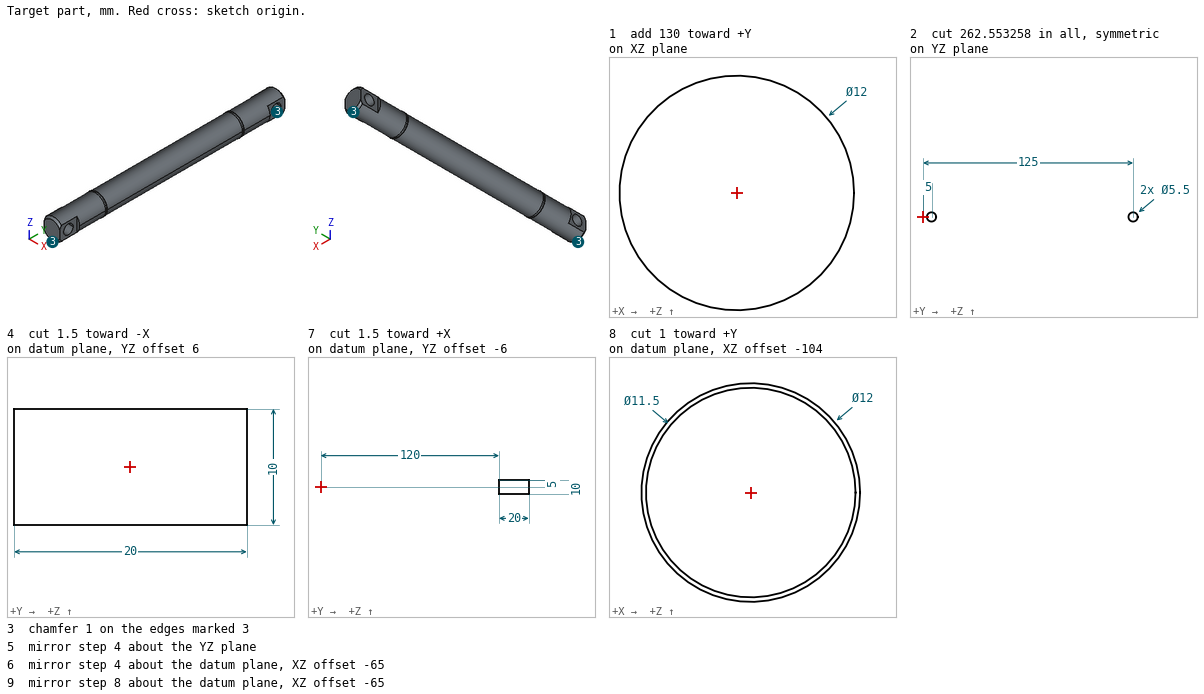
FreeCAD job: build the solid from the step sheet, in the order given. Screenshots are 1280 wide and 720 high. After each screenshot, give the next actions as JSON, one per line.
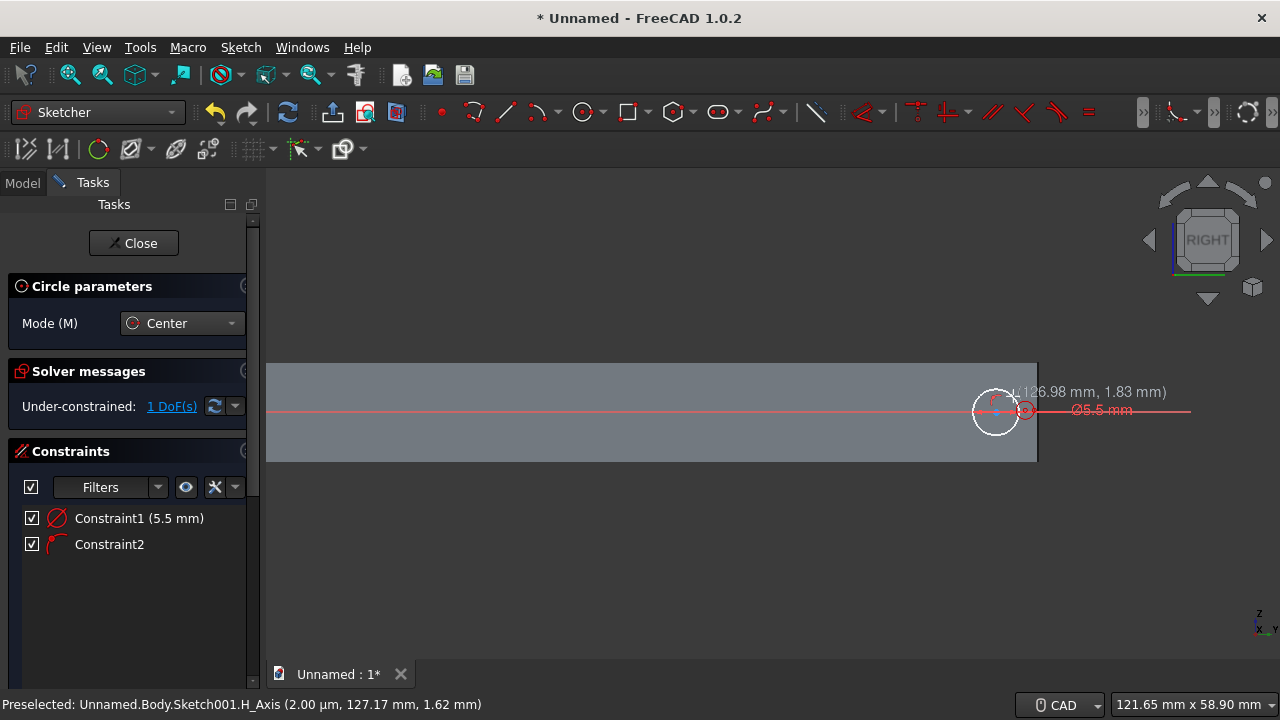
{"action": "scroll", "coordinate": [969, 415], "scroll_direction": "down", "scroll_amount": 3}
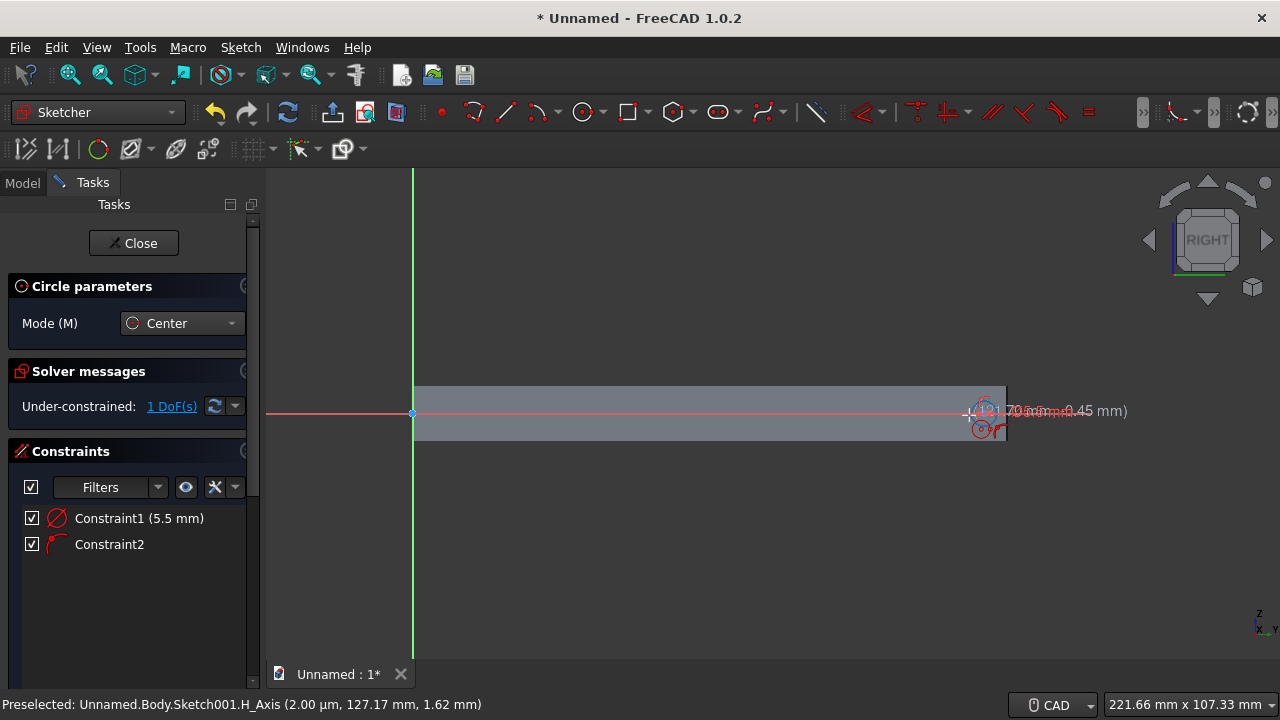
{"action": "scroll", "coordinate": [435, 414], "scroll_direction": "up", "scroll_amount": 3}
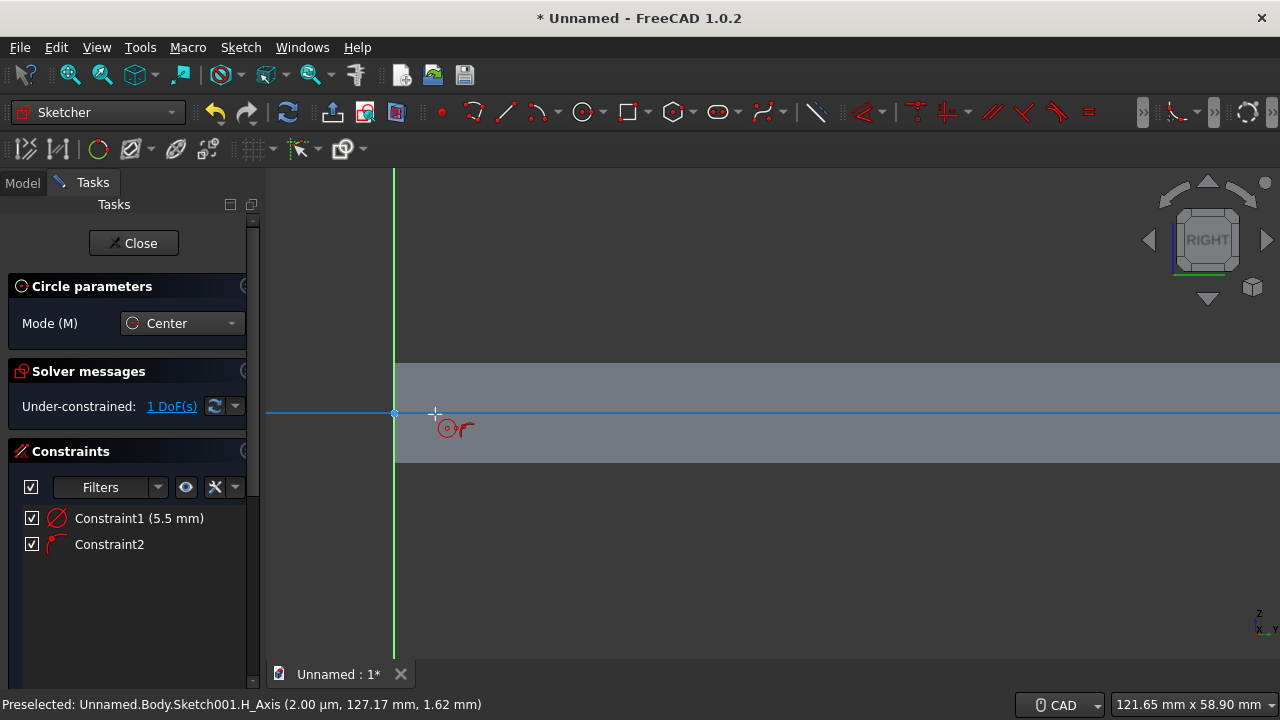
{"action": "left_click", "coordinate": [436, 413]}
{"action": "mouse_move", "coordinate": [452, 397]}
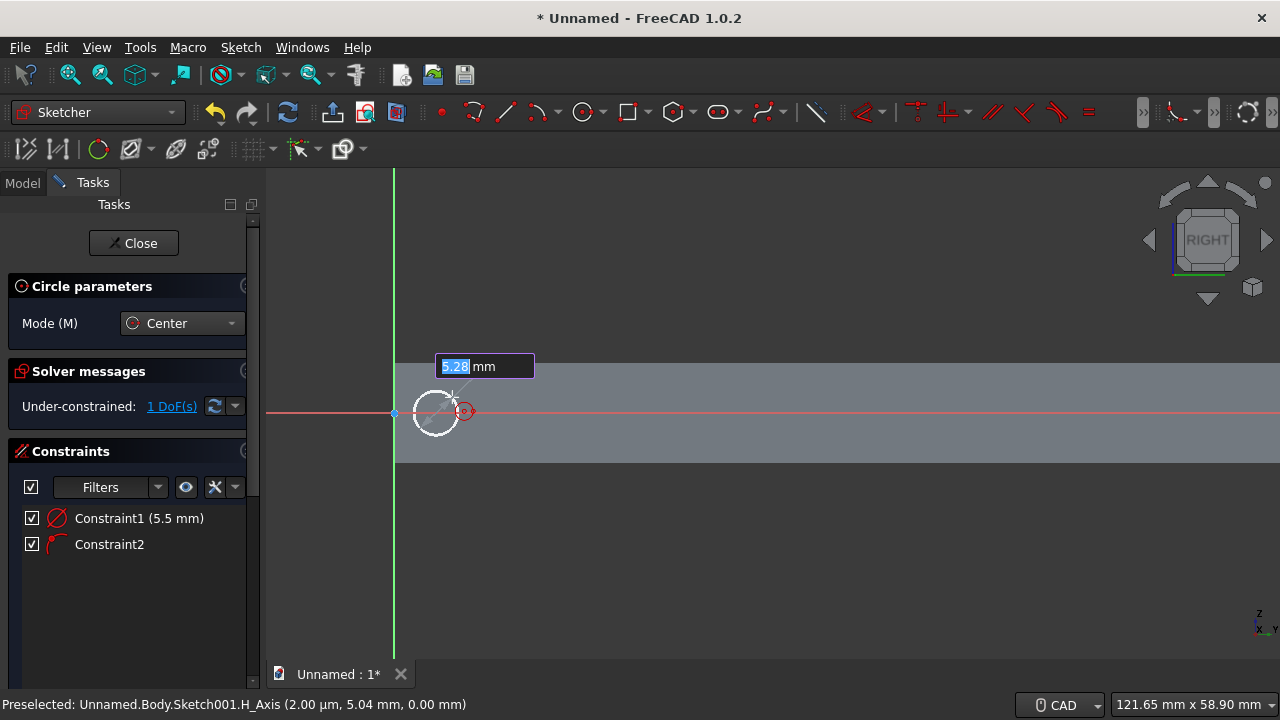
{"action": "type", "text": "5.5"}
{"action": "key", "text": "Return"}
{"action": "key", "text": "Escape"}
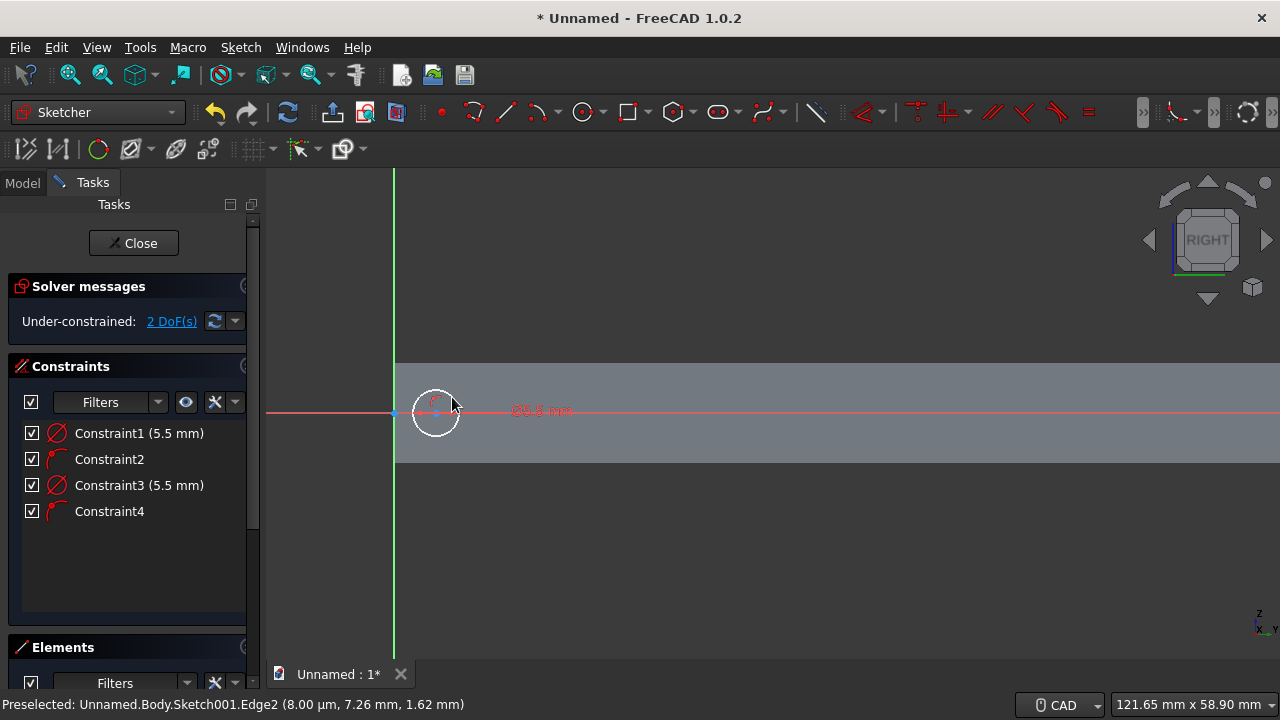
{"action": "key", "text": "d"}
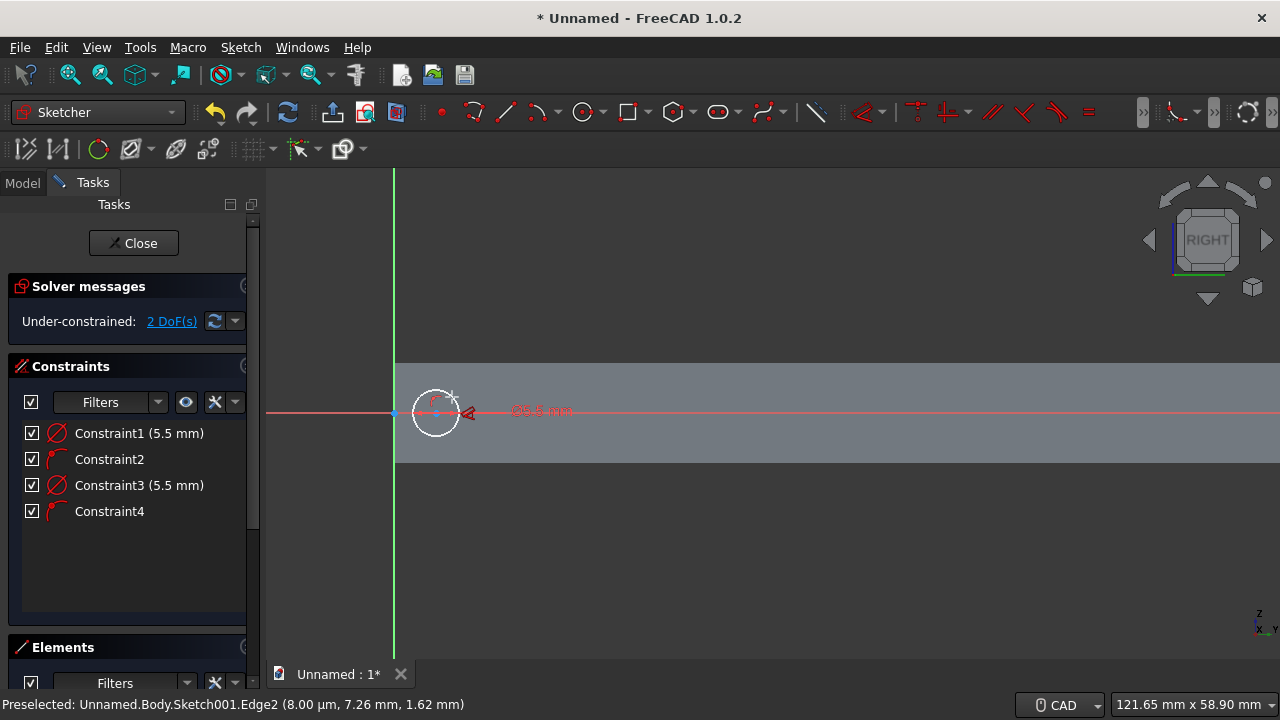
{"action": "left_click", "coordinate": [436, 413]}
{"action": "left_click", "coordinate": [415, 447]}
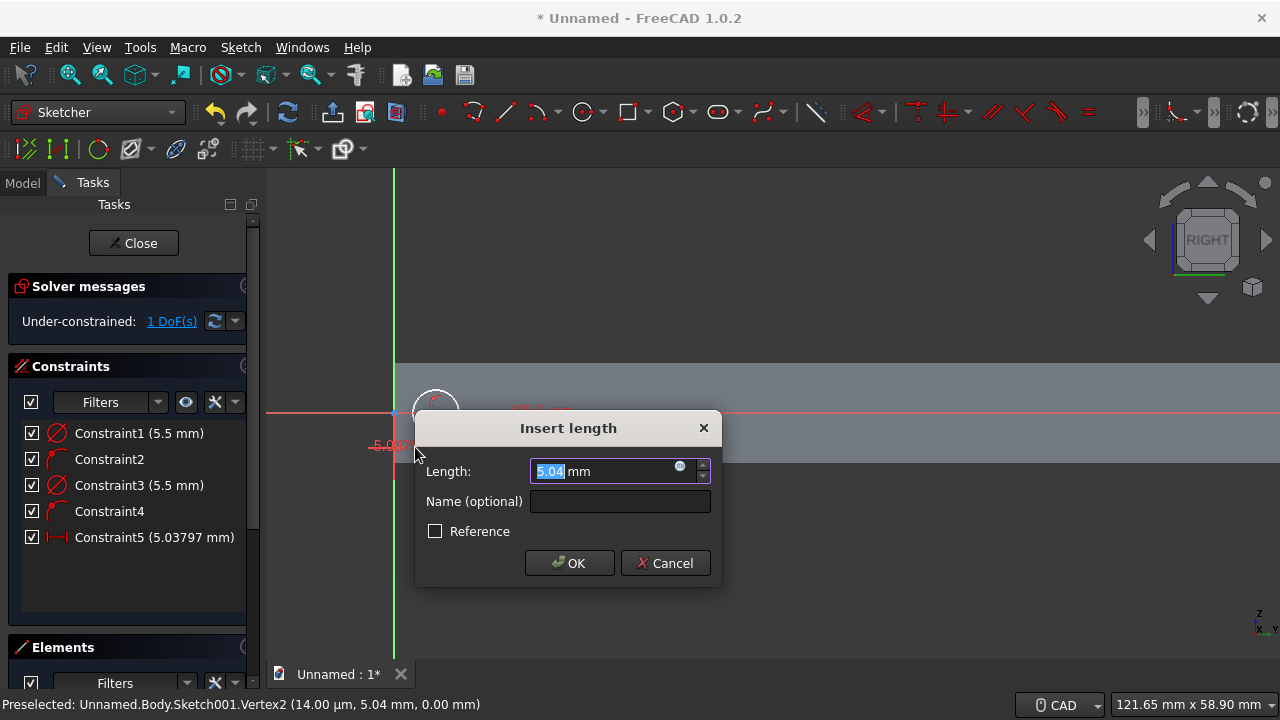
{"action": "type", "text": "5"}
{"action": "key", "text": "Return"}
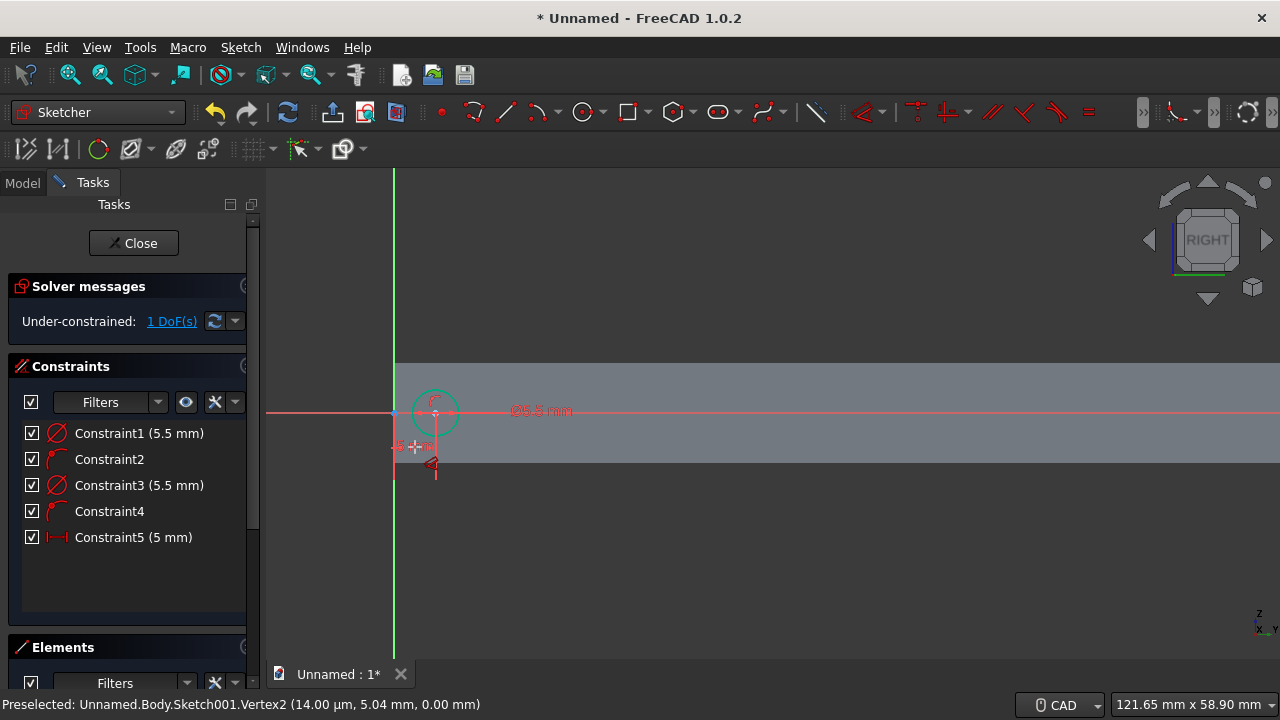
{"action": "scroll", "coordinate": [435, 414], "scroll_direction": "down", "scroll_amount": 3}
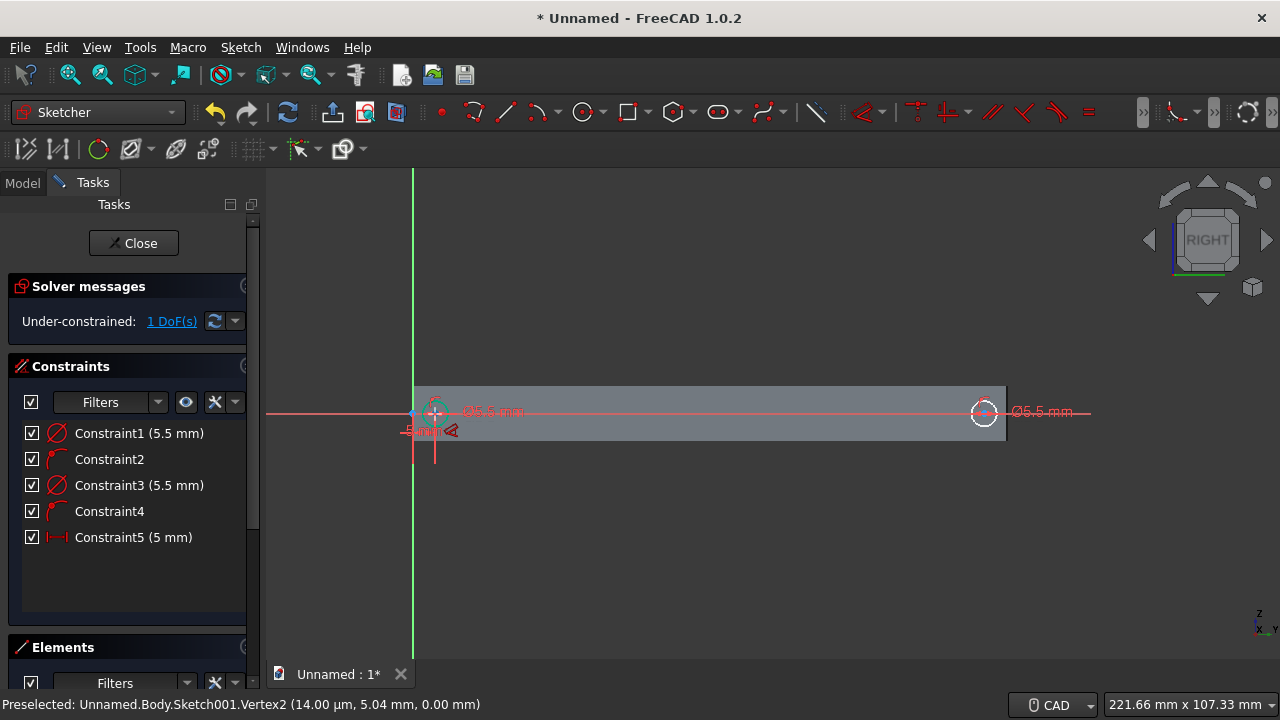
{"action": "left_click", "coordinate": [984, 414]}
{"action": "left_click", "coordinate": [698, 448]}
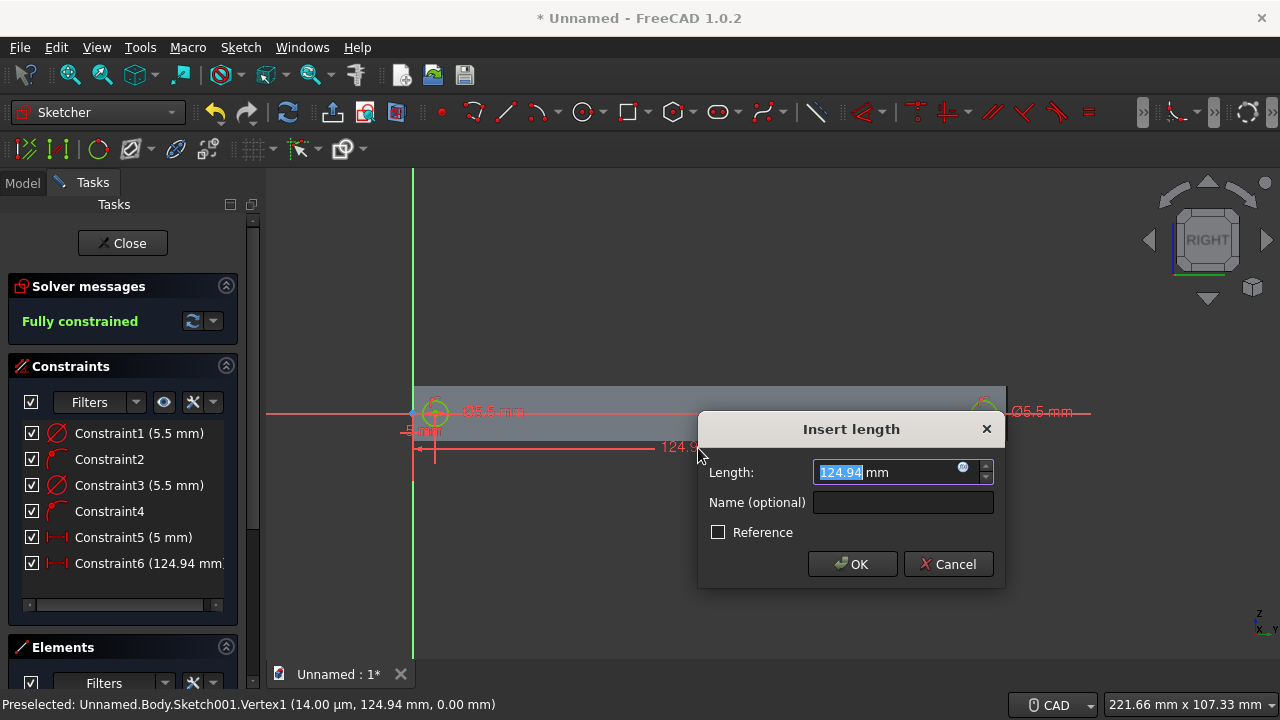
{"action": "type", "text": "125"}
{"action": "key", "text": "Return"}
{"action": "key", "text": "Escape"}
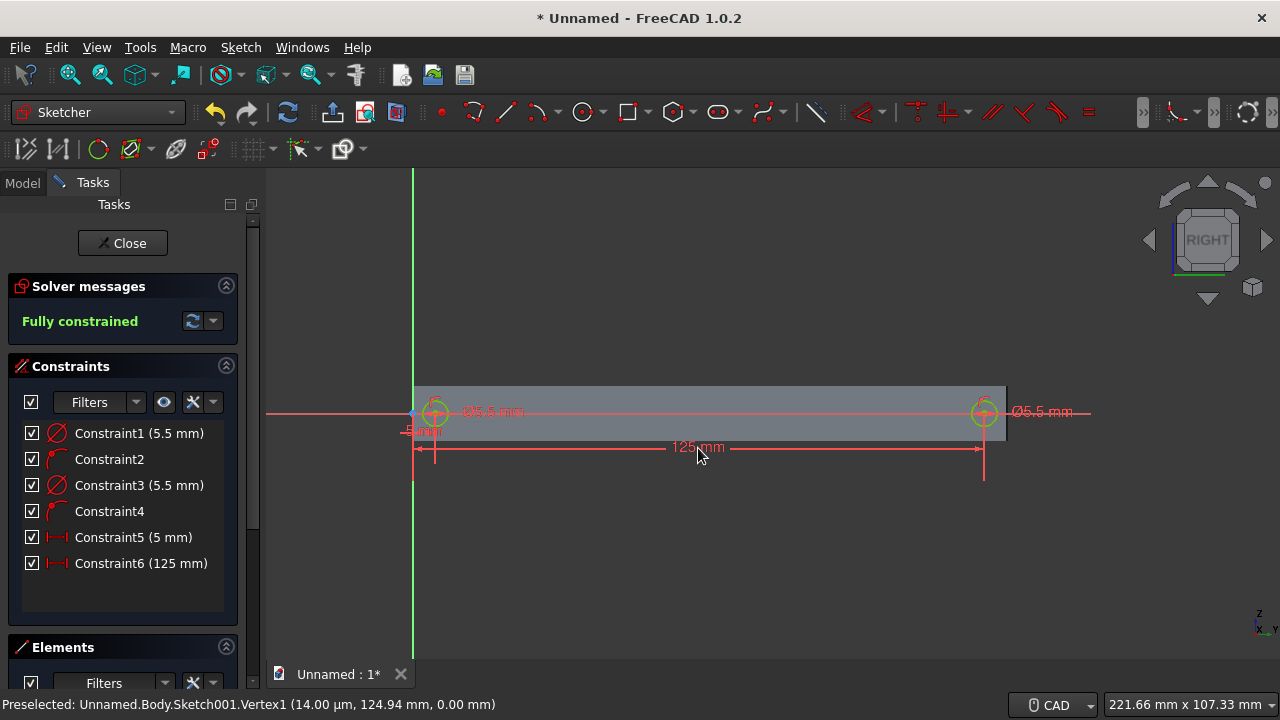
{"action": "left_click", "coordinate": [123, 243]}